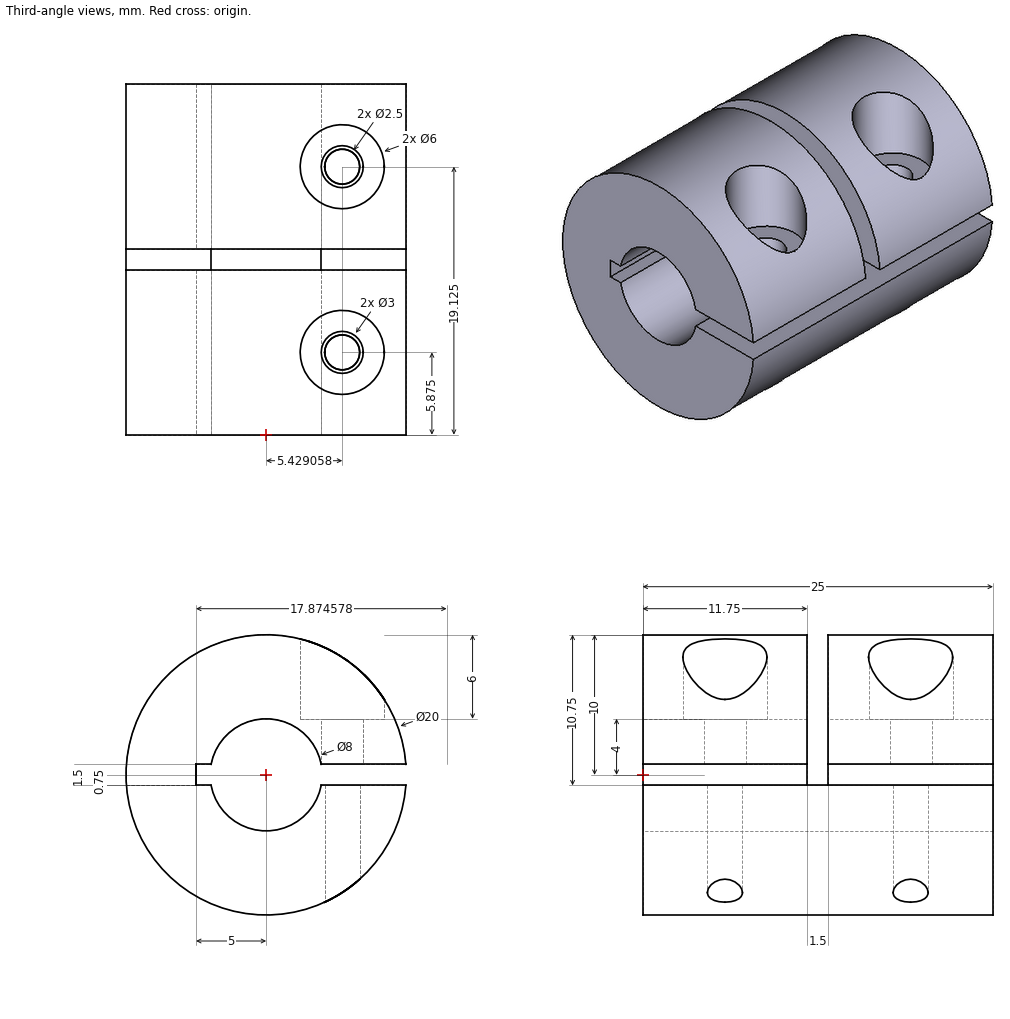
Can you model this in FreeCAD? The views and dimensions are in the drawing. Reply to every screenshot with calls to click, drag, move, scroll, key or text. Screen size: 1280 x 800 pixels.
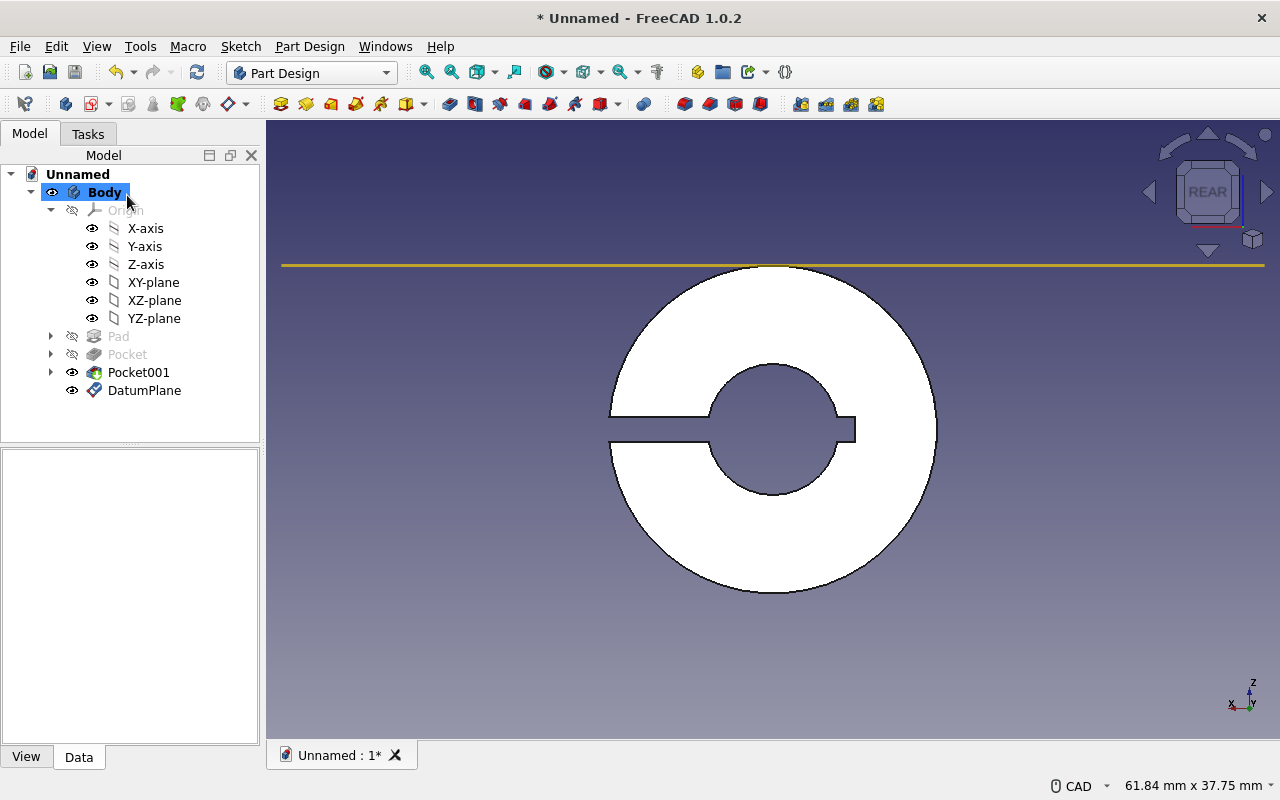
click(117, 390)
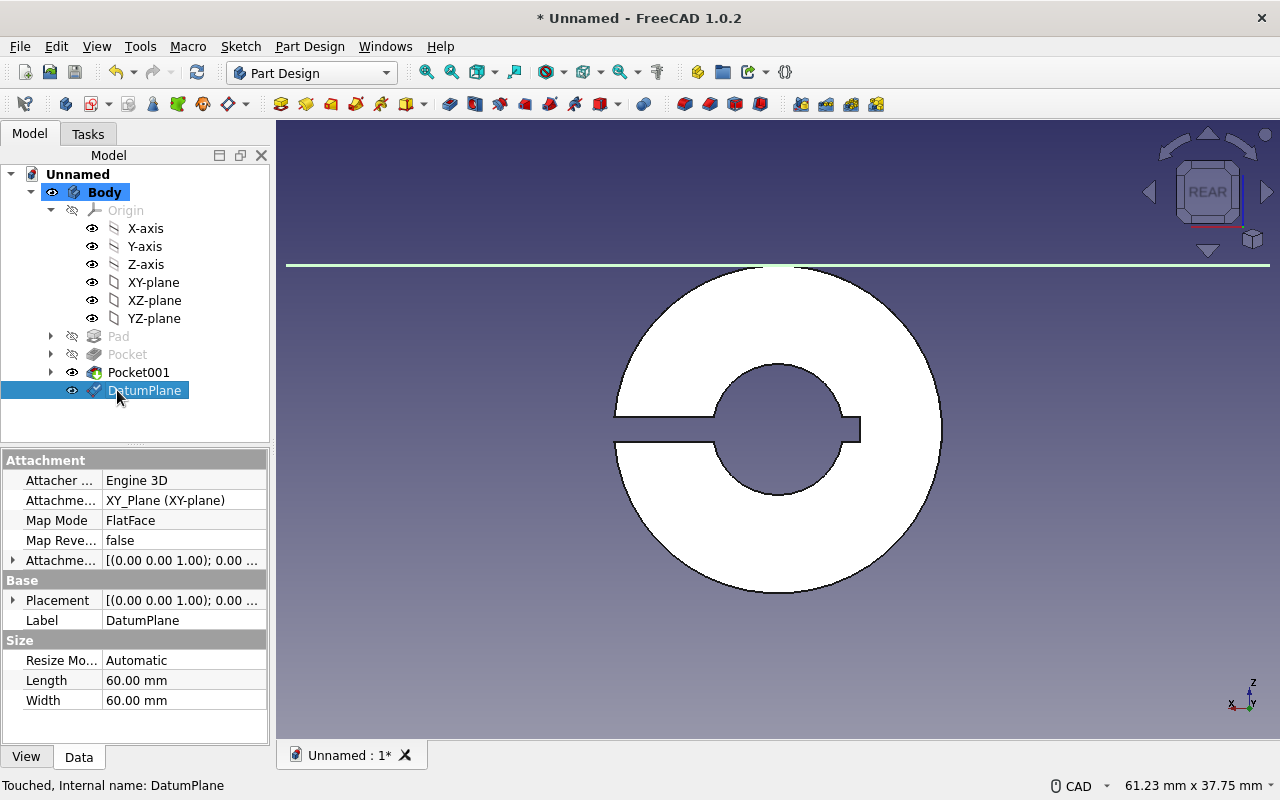
click(90, 104)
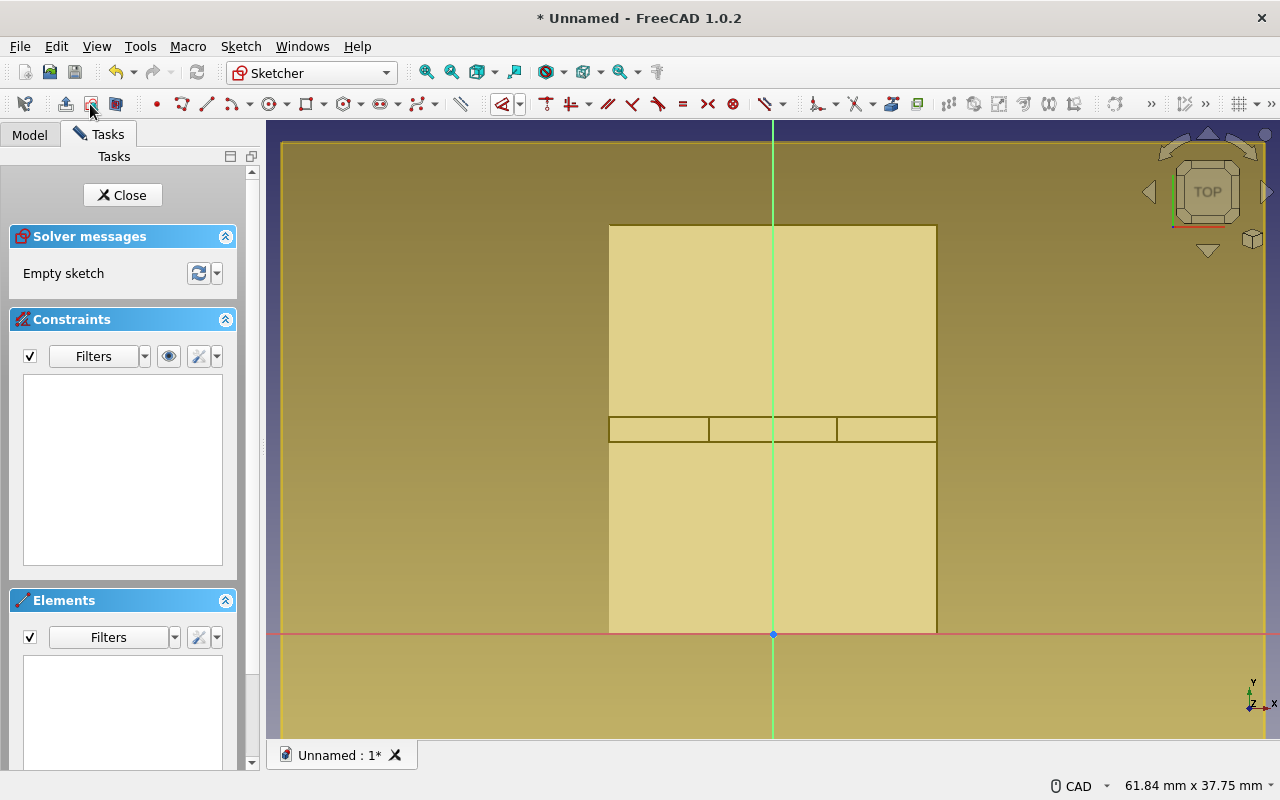
click(268, 104)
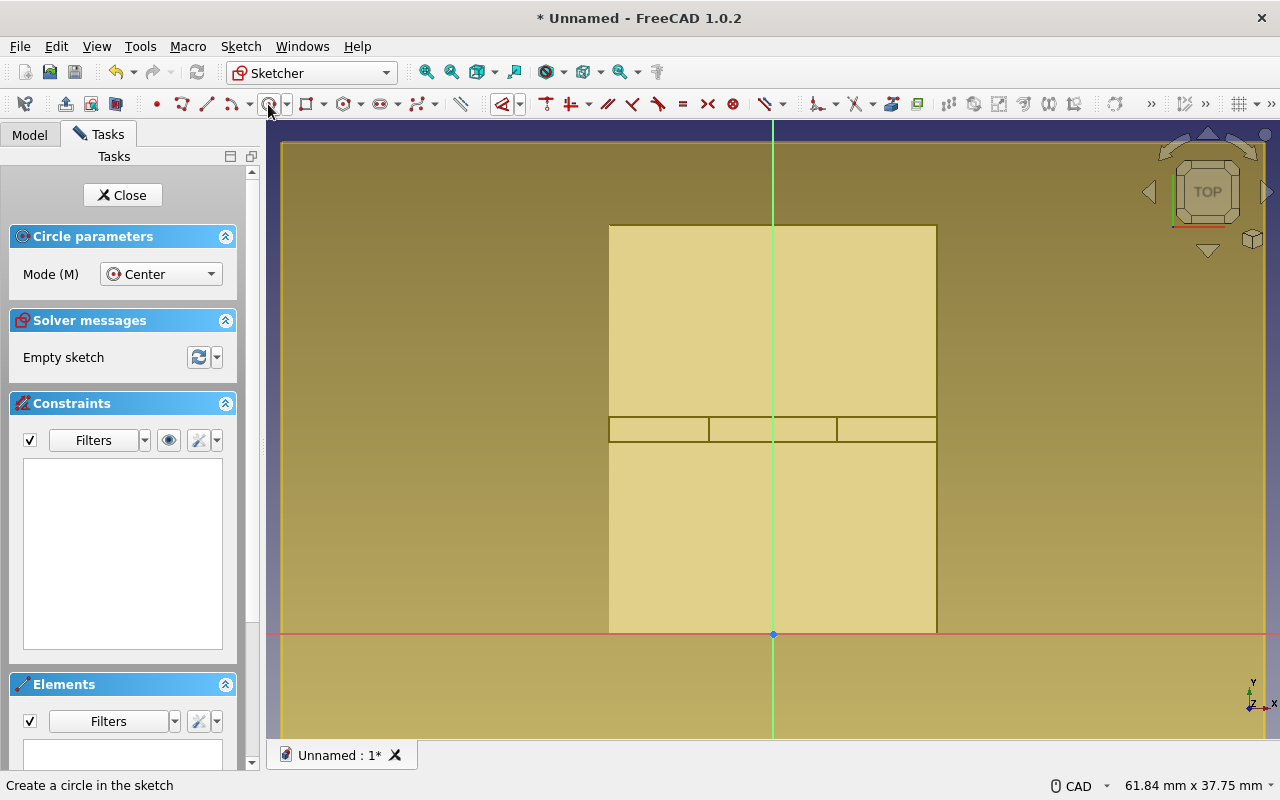
click(862, 321)
click(897, 286)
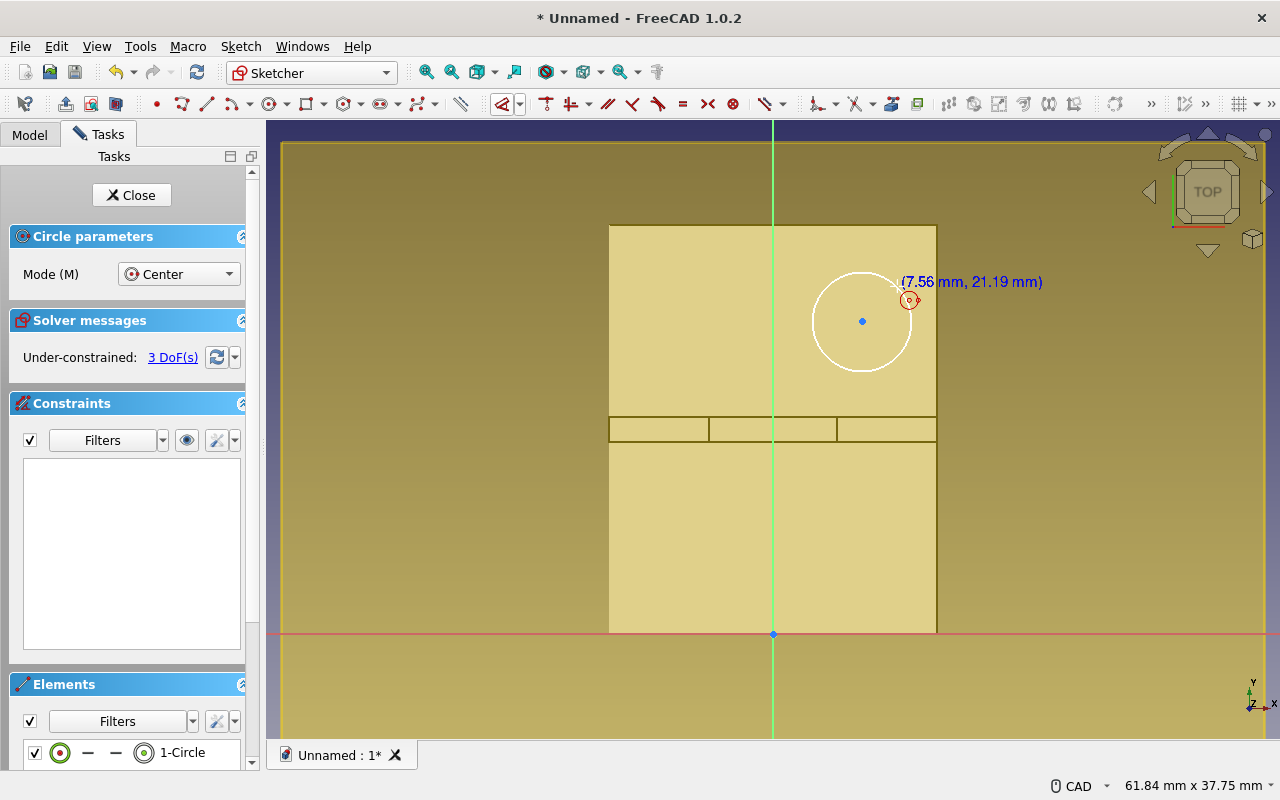
click(862, 538)
click(897, 503)
key(Escape)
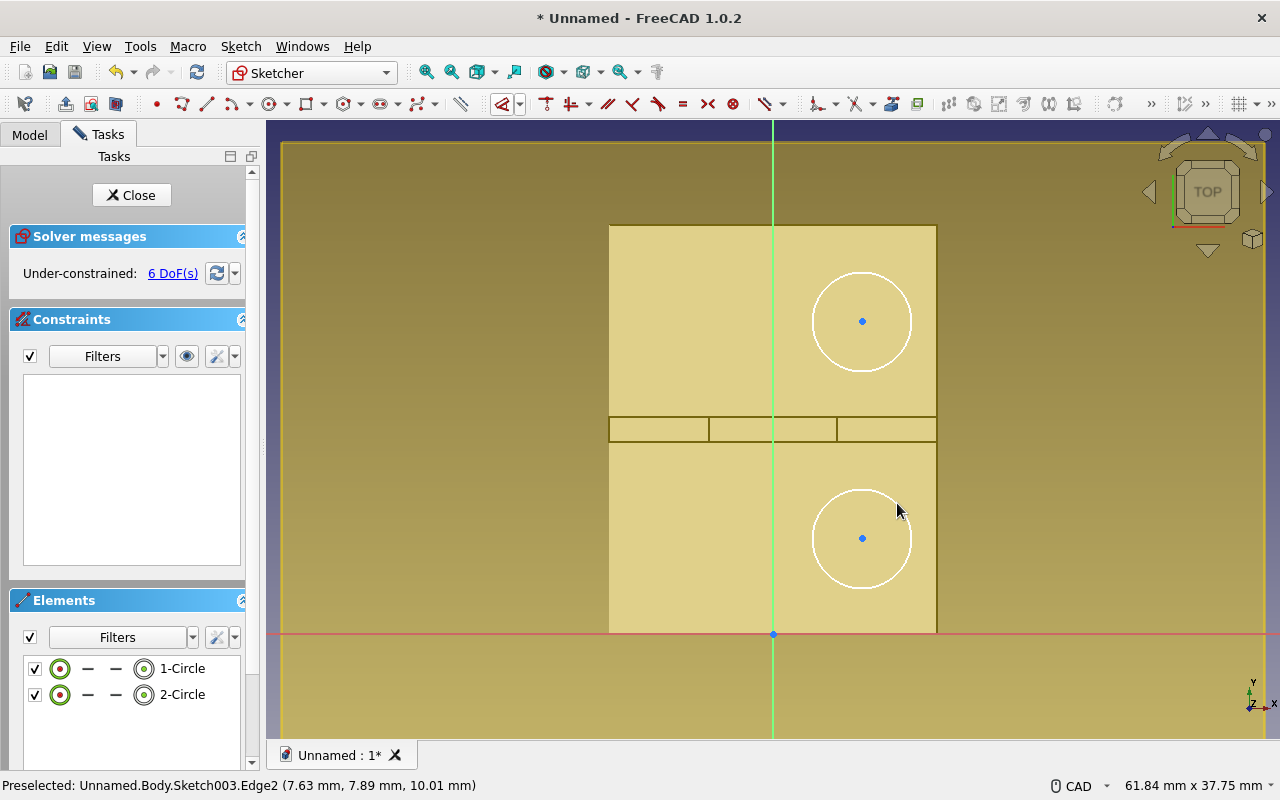
click(897, 287)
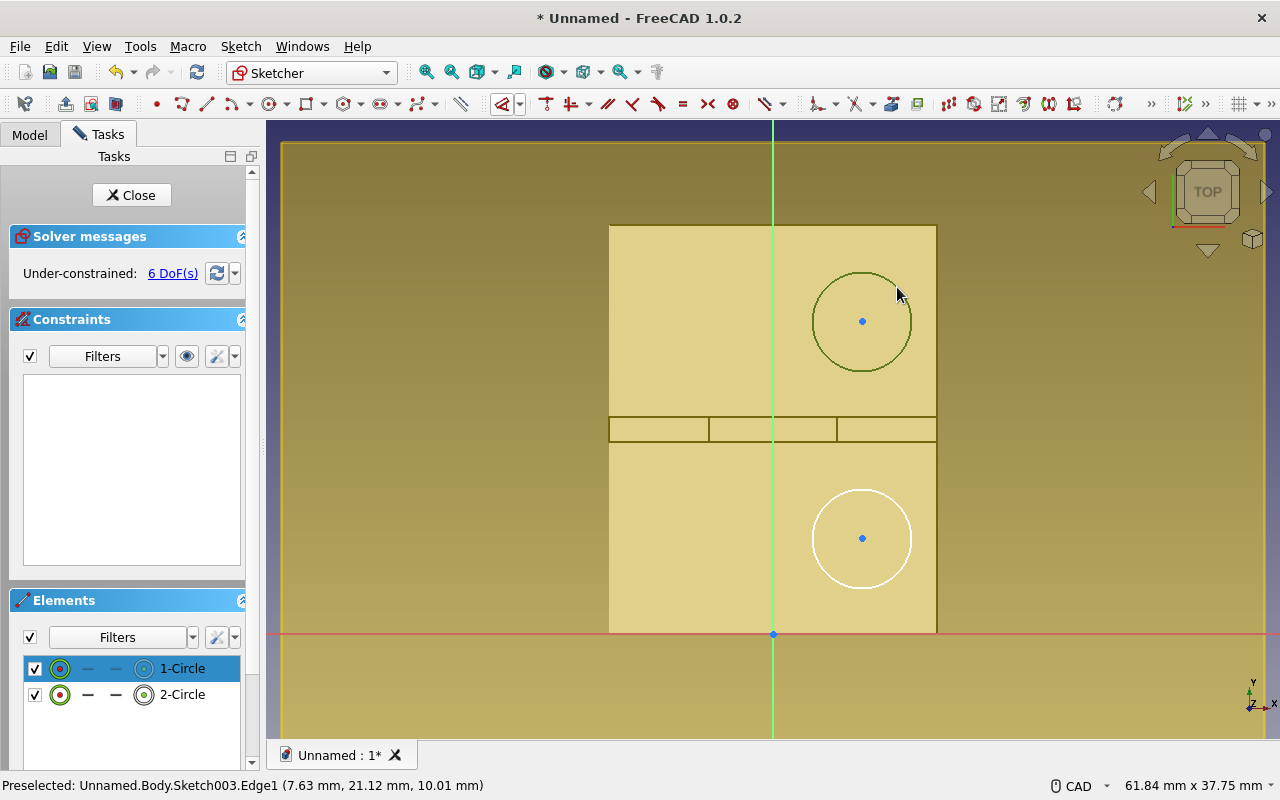
click(897, 504)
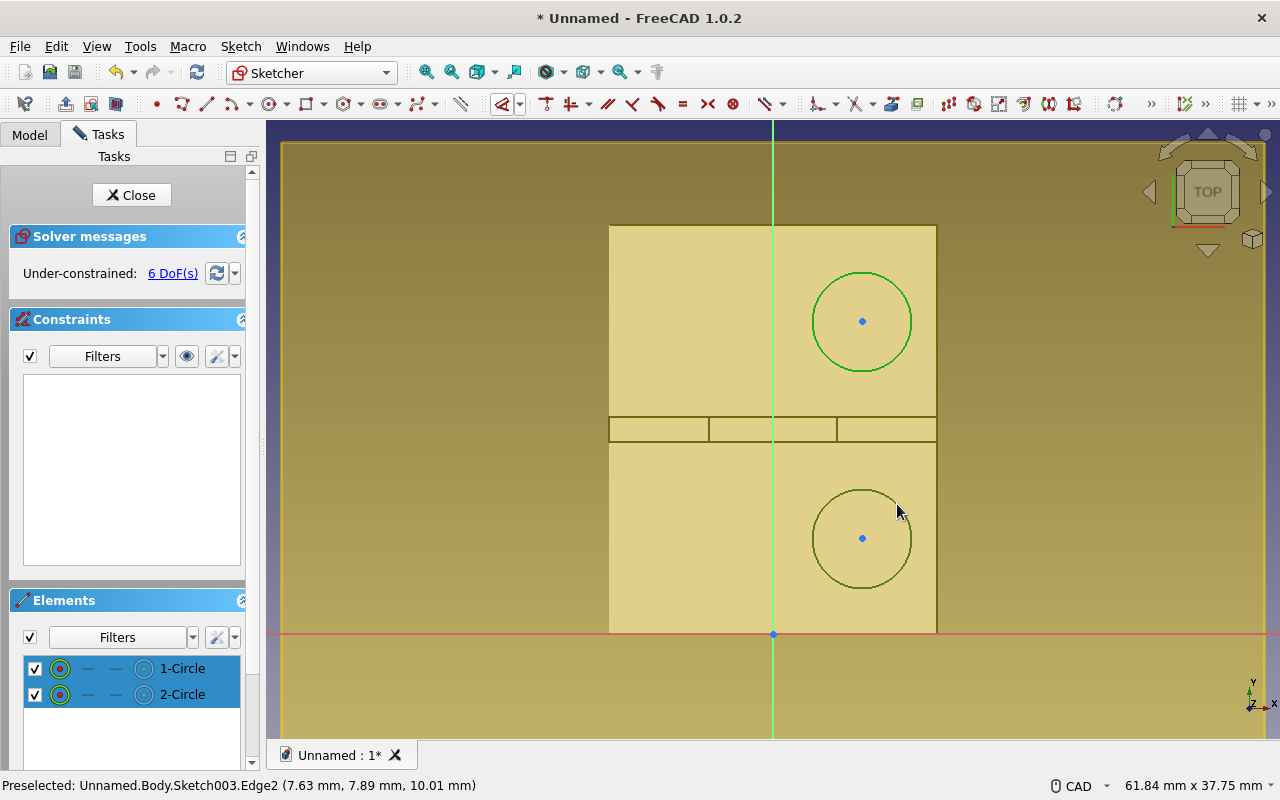
click(683, 104)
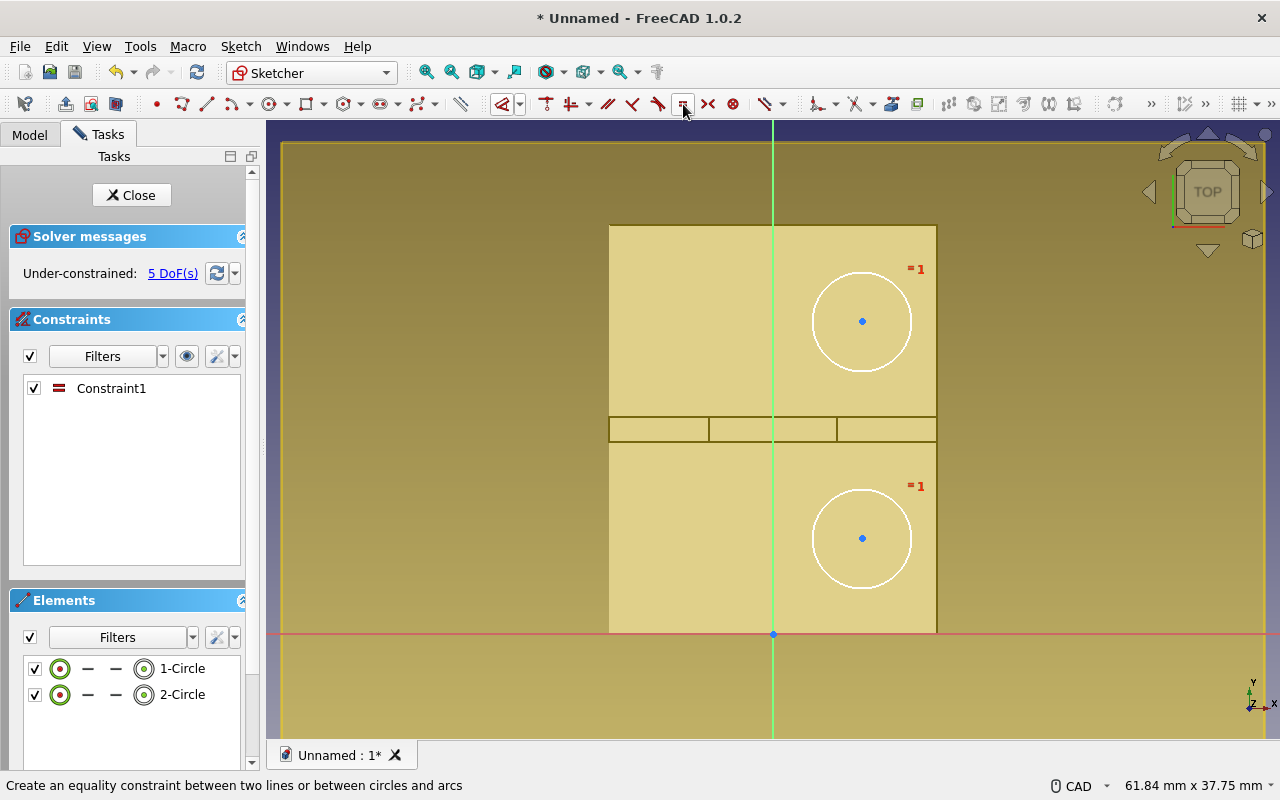
click(862, 322)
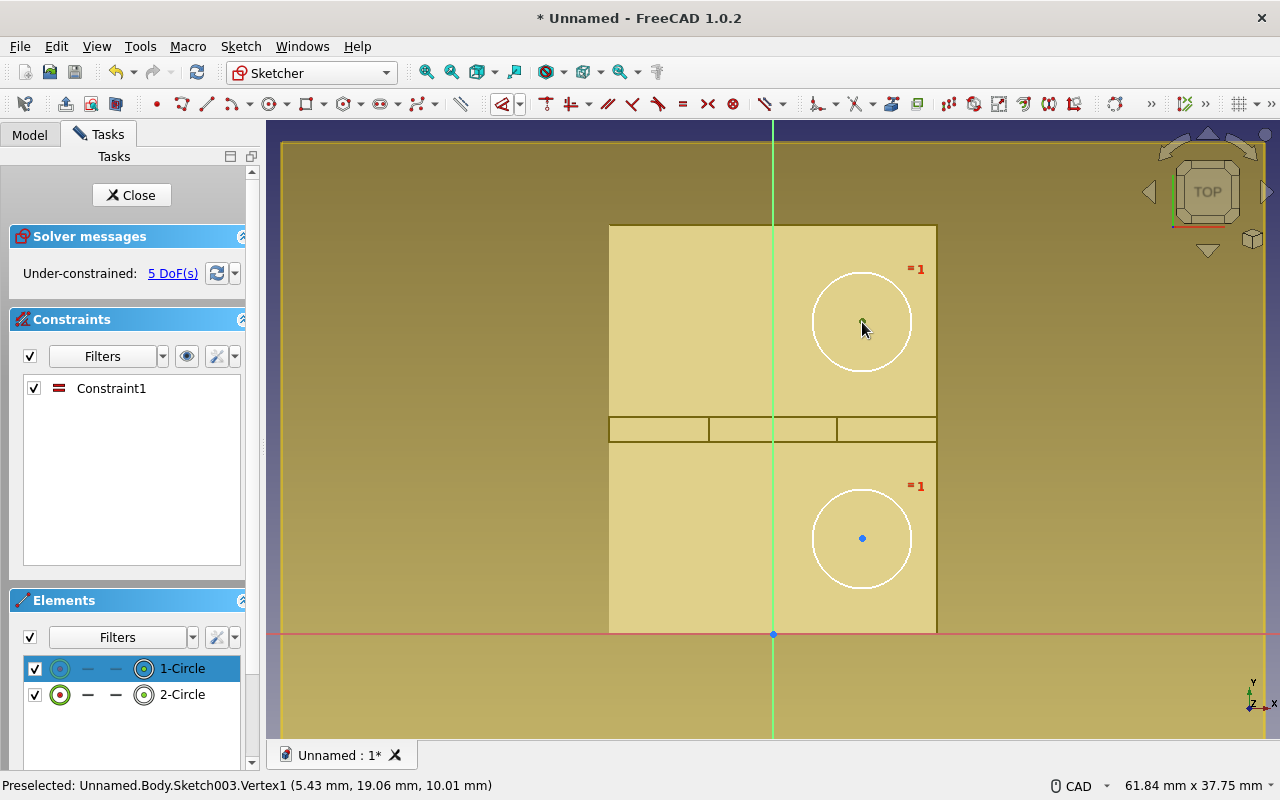
click(862, 539)